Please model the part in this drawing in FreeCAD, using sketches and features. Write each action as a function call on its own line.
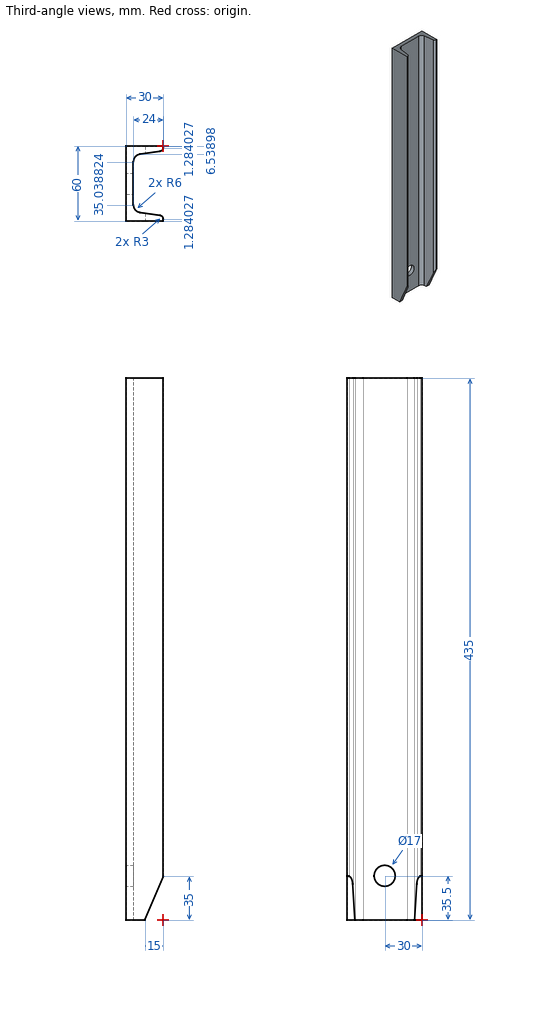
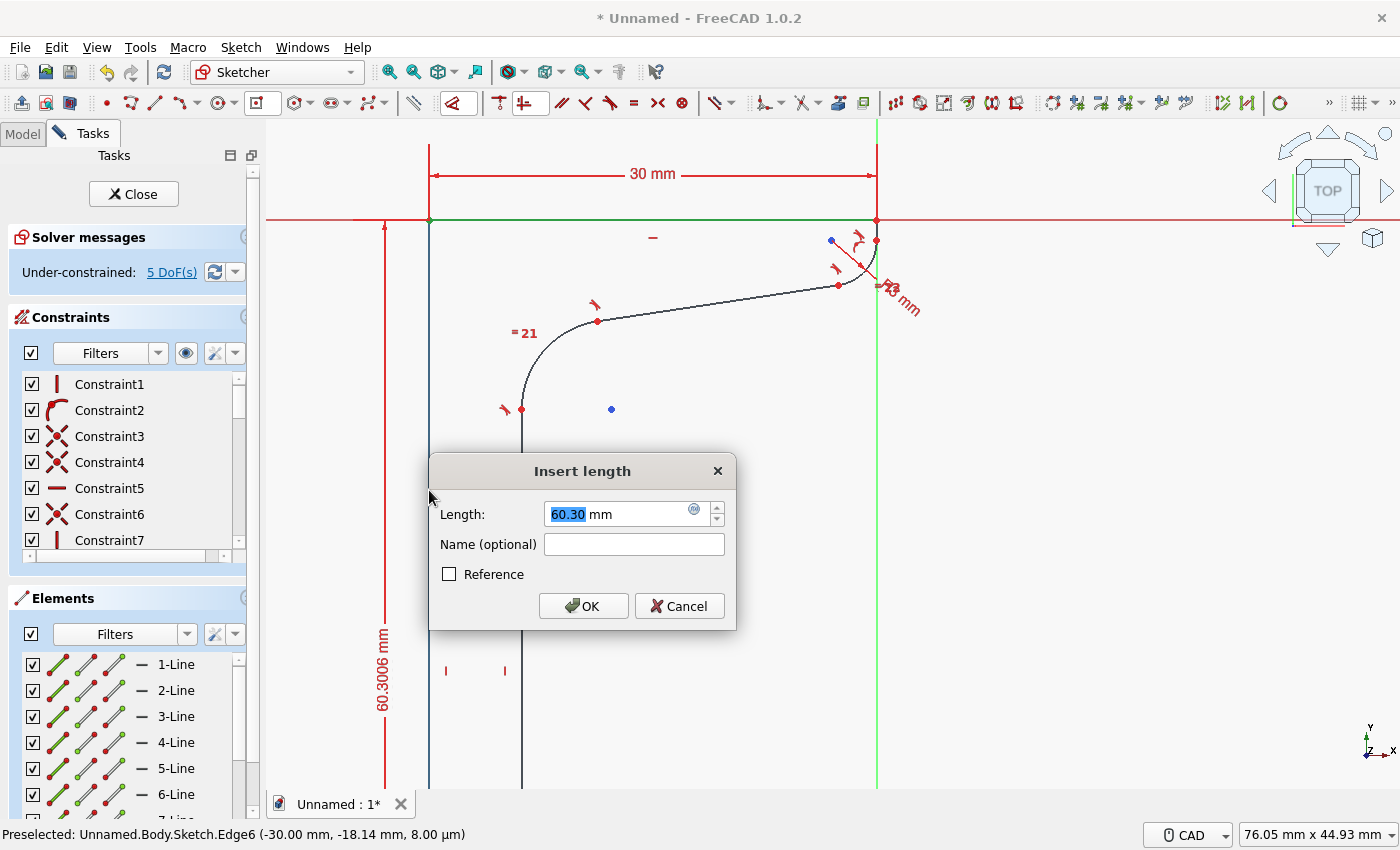
text(60)
key(Return)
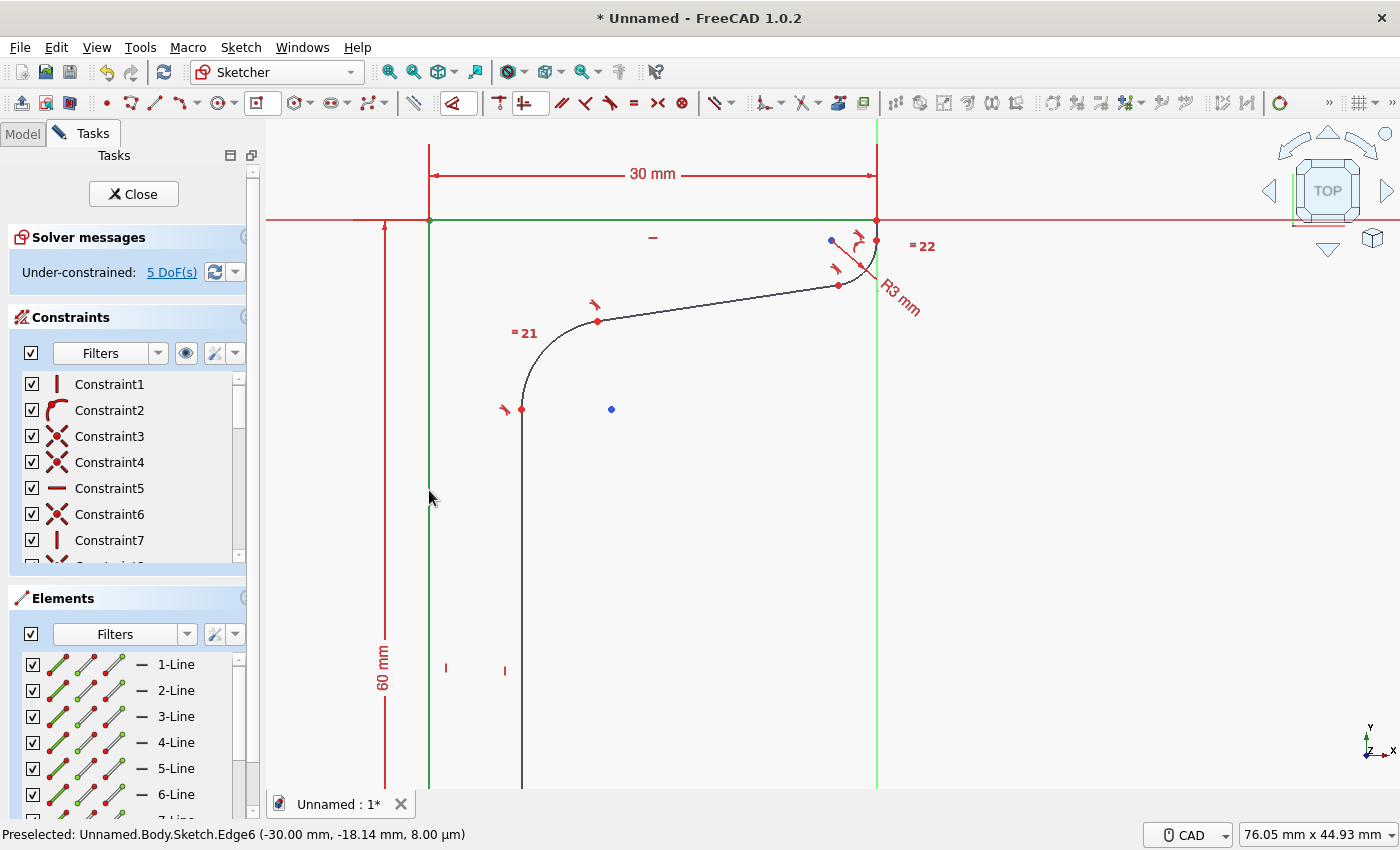
scroll(855, 280, down, 4)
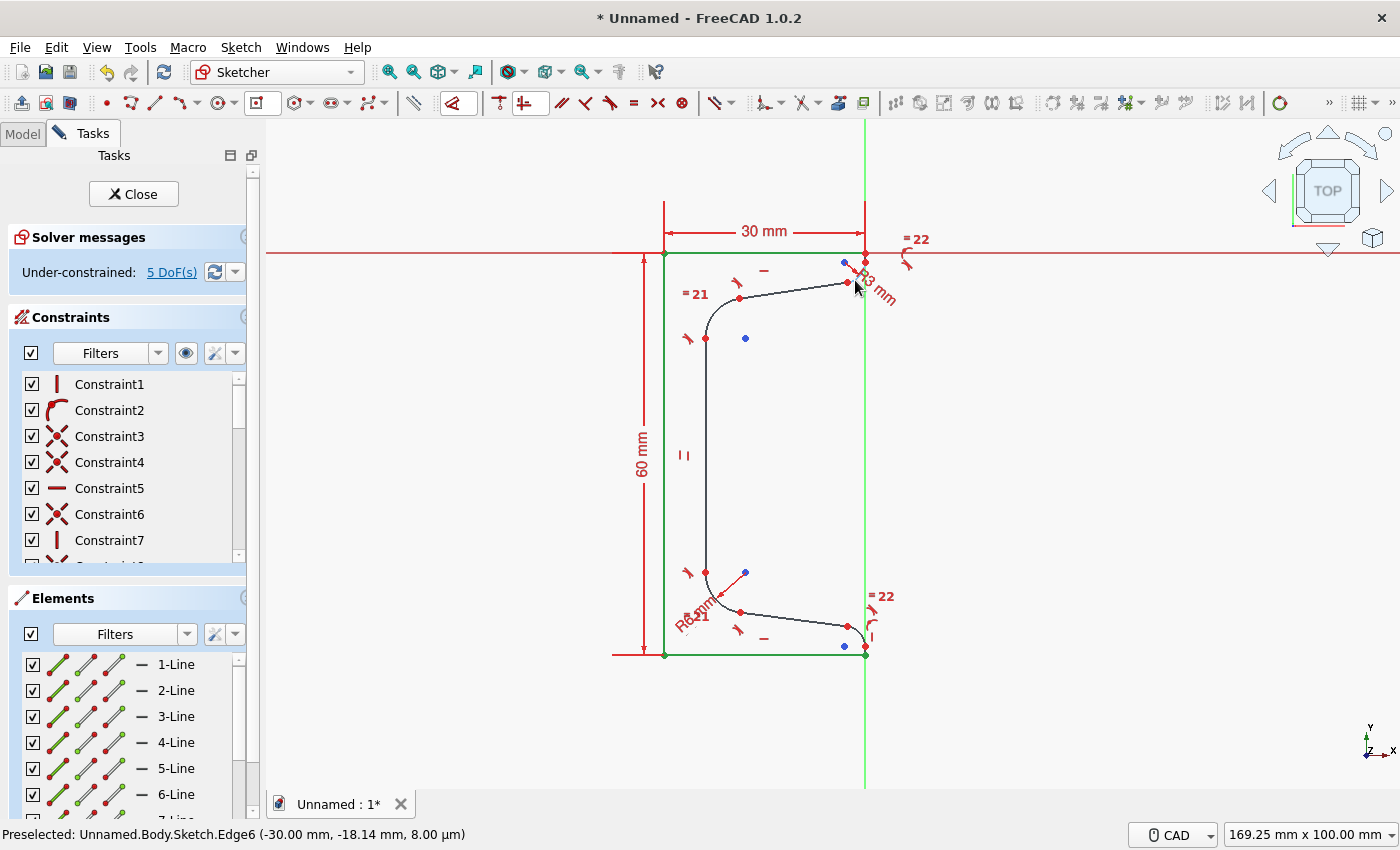
click(706, 573)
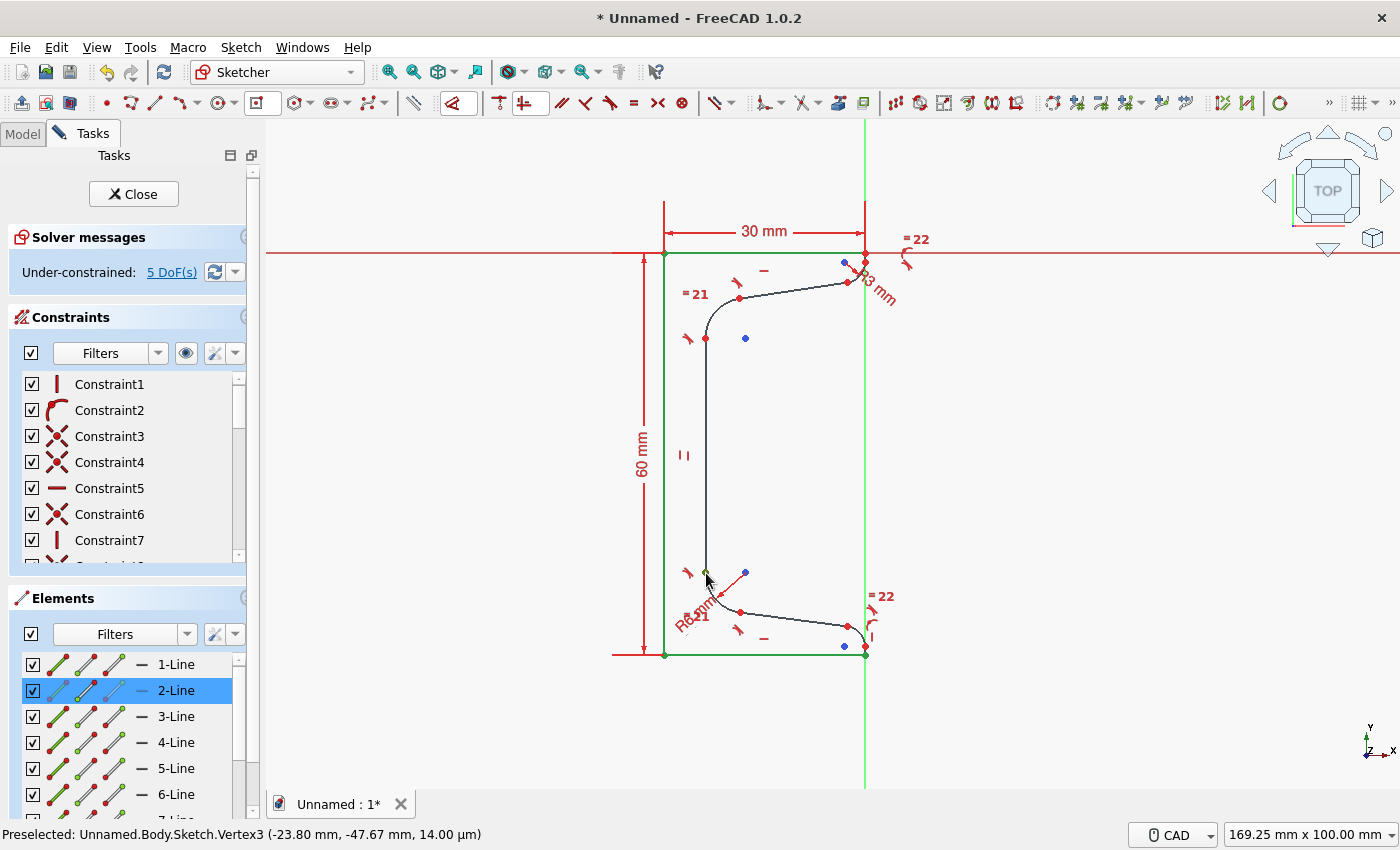
key(l)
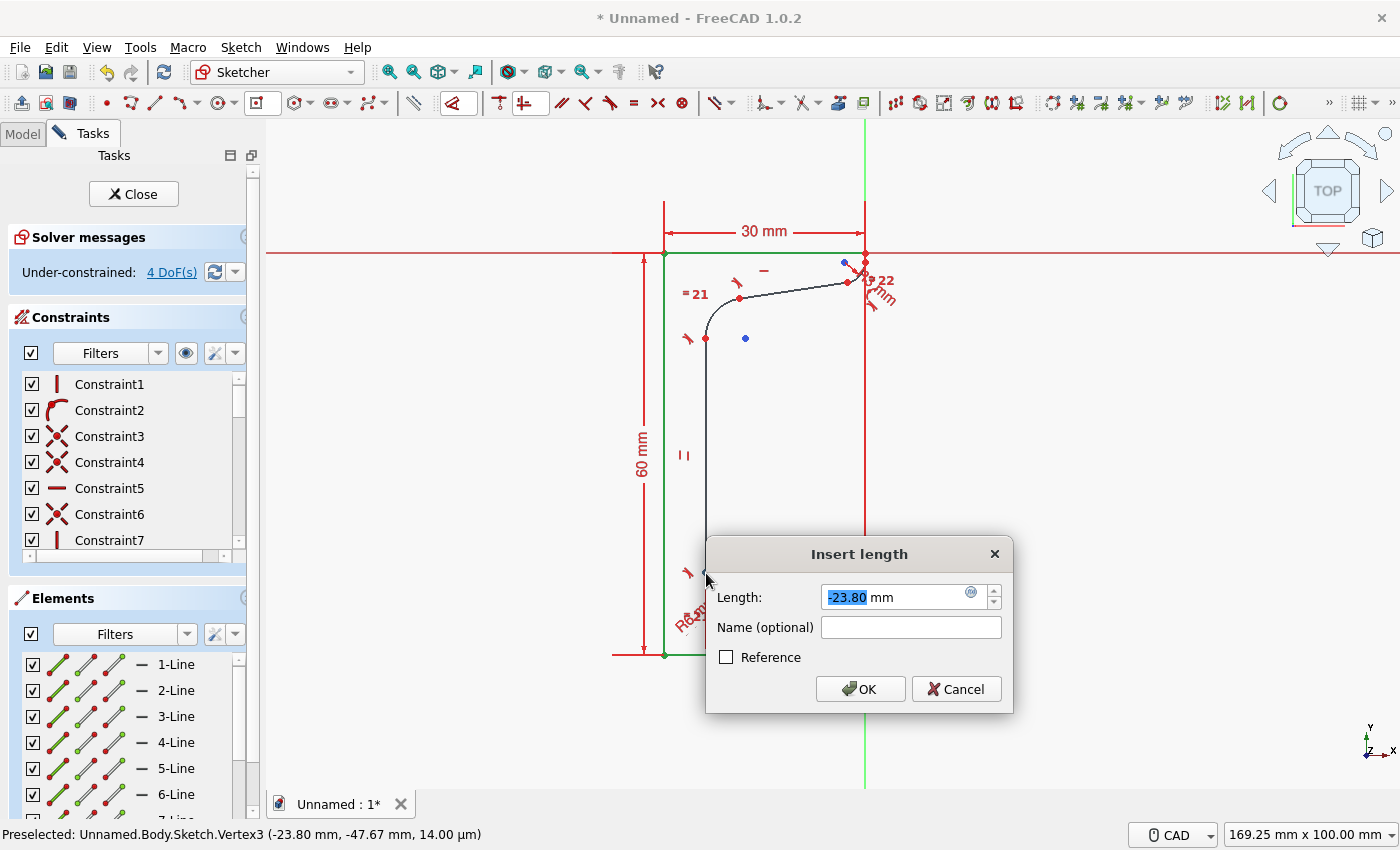
text(-24)
key(Return)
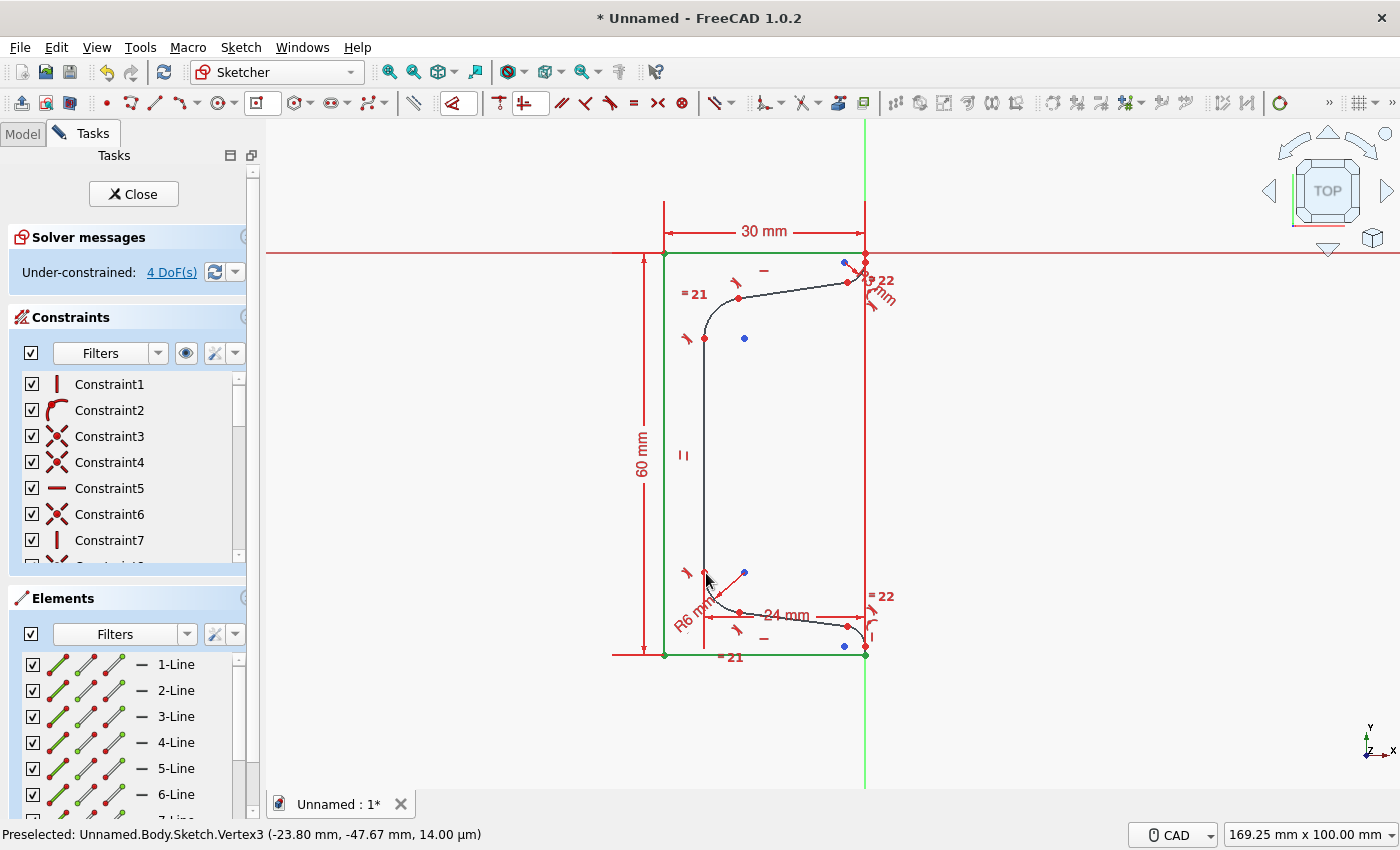
scroll(865, 258, up, 8)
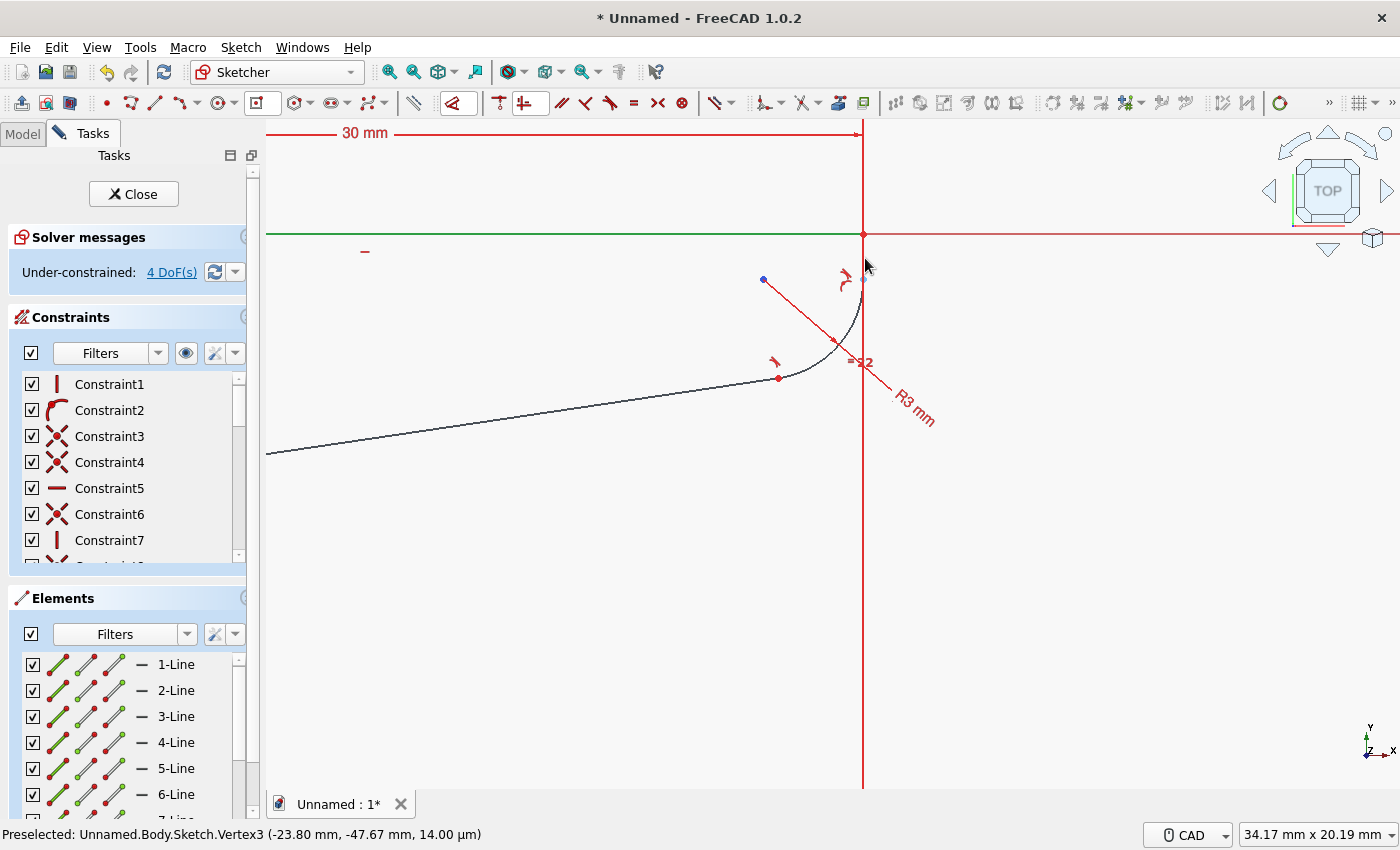
click(863, 257)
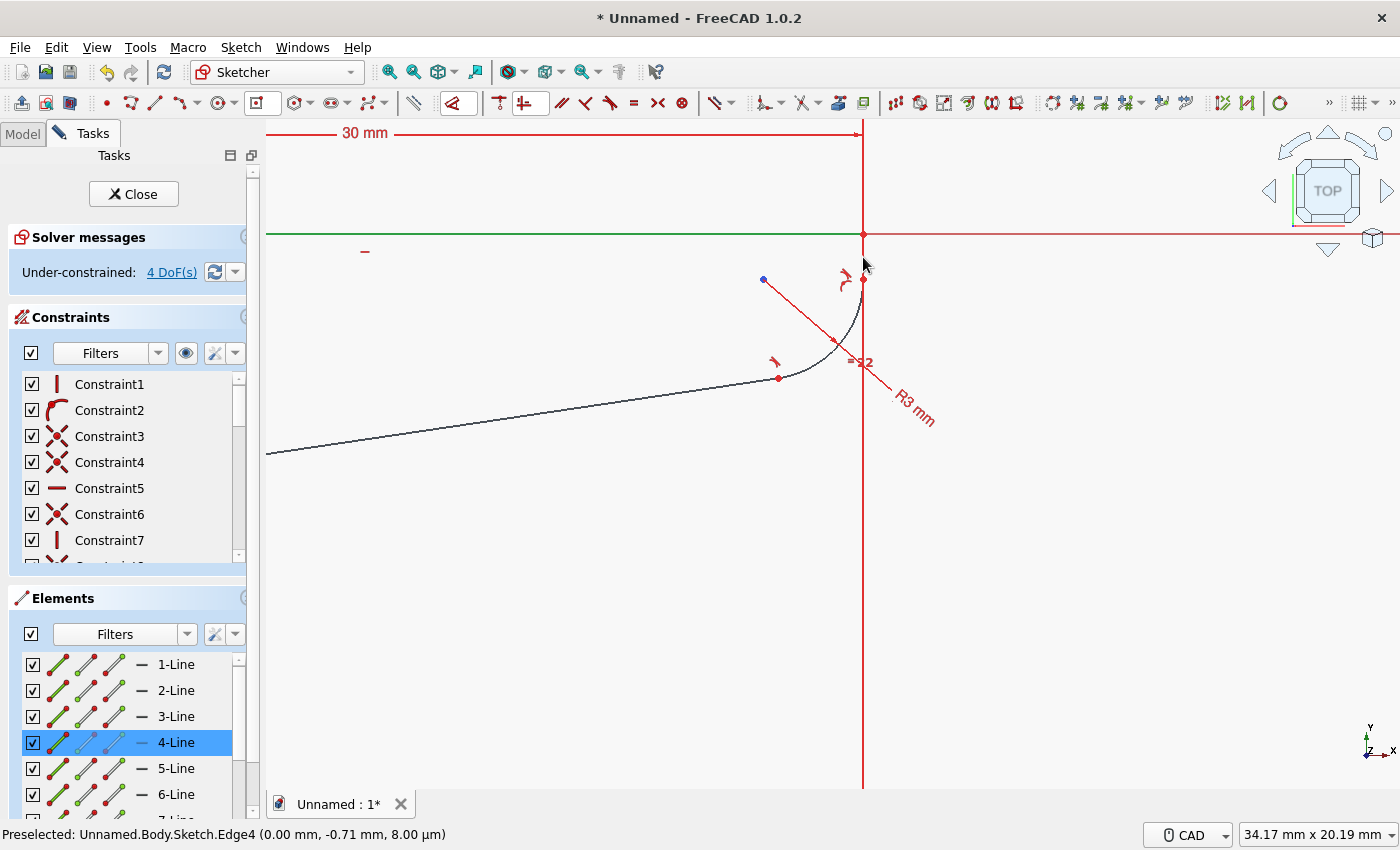
key(i)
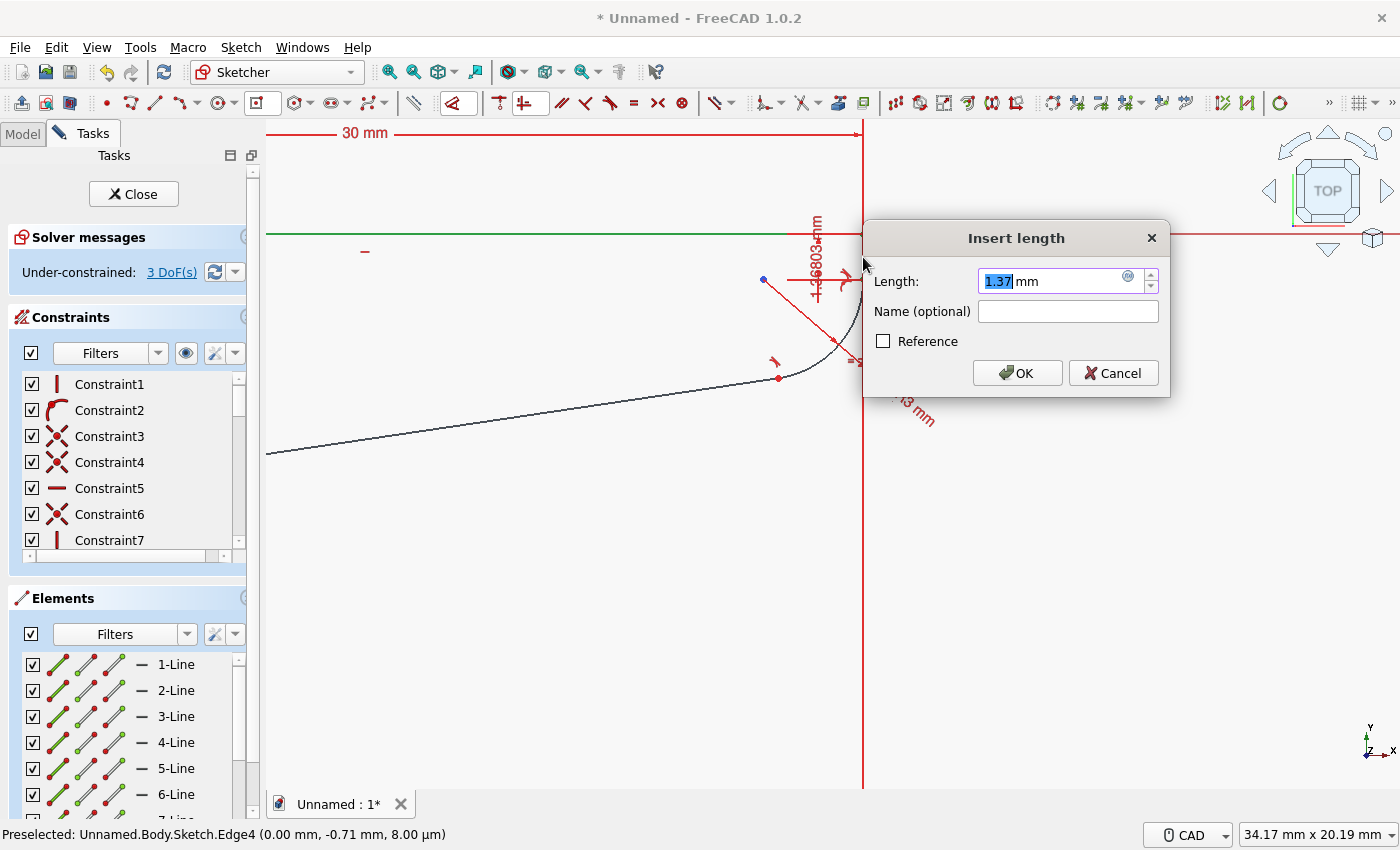
text(1.284027)
key(Return)